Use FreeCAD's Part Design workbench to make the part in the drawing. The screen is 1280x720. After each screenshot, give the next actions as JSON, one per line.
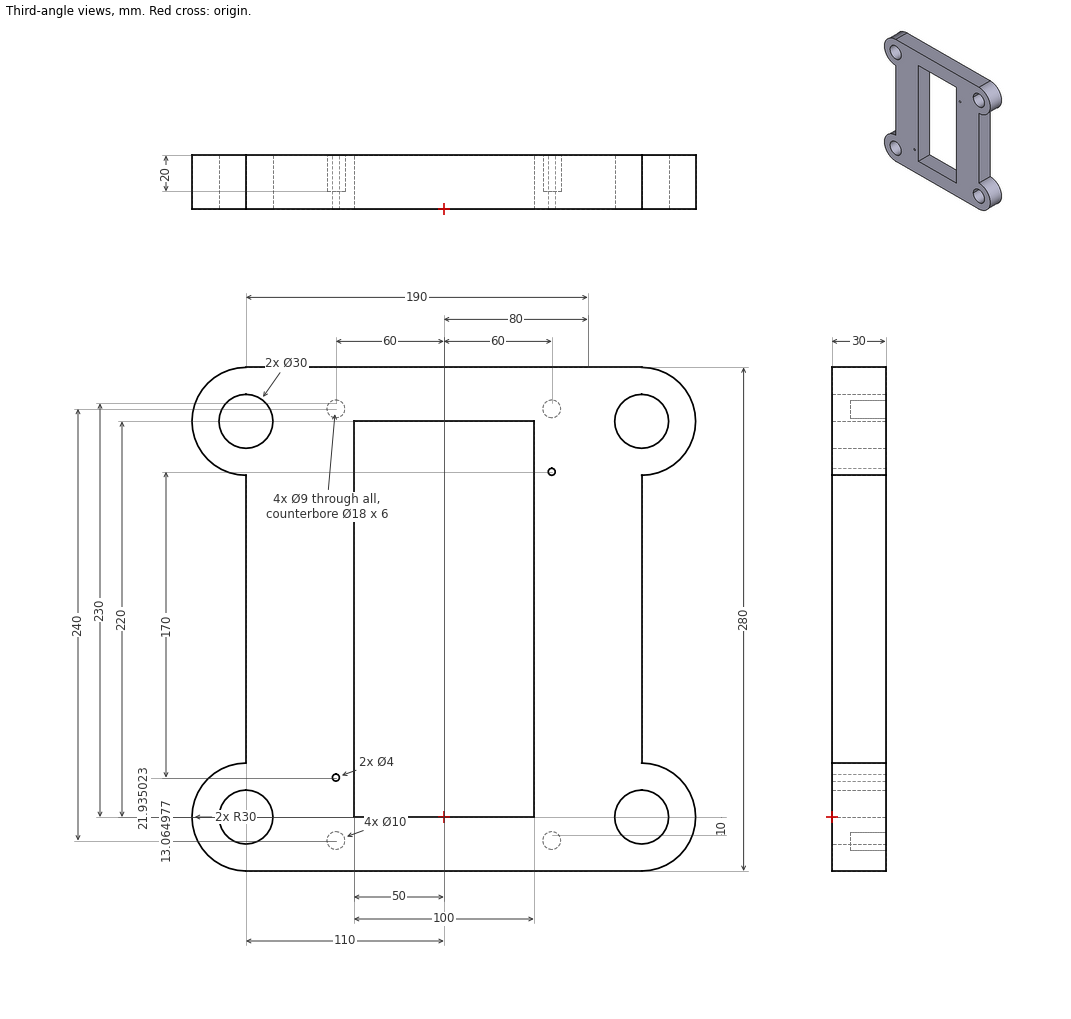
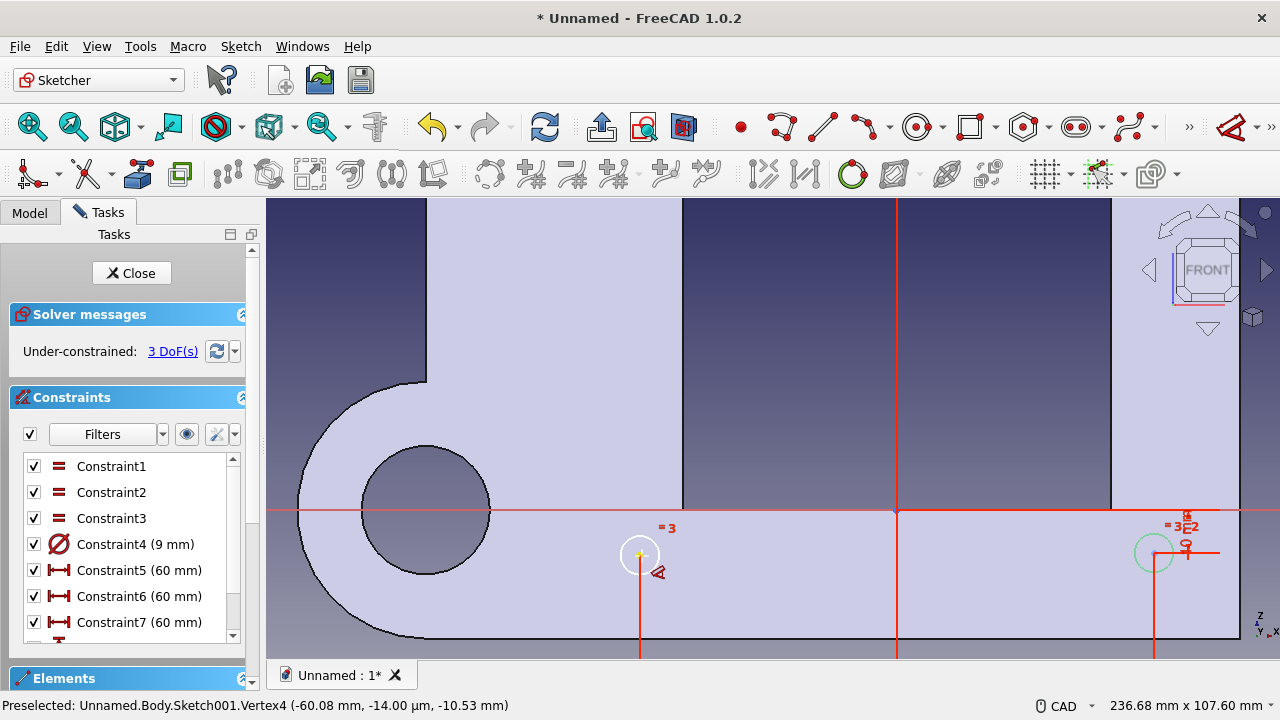
{"action": "left_click", "coordinate": [640, 555]}
{"action": "left_click", "coordinate": [606, 533]}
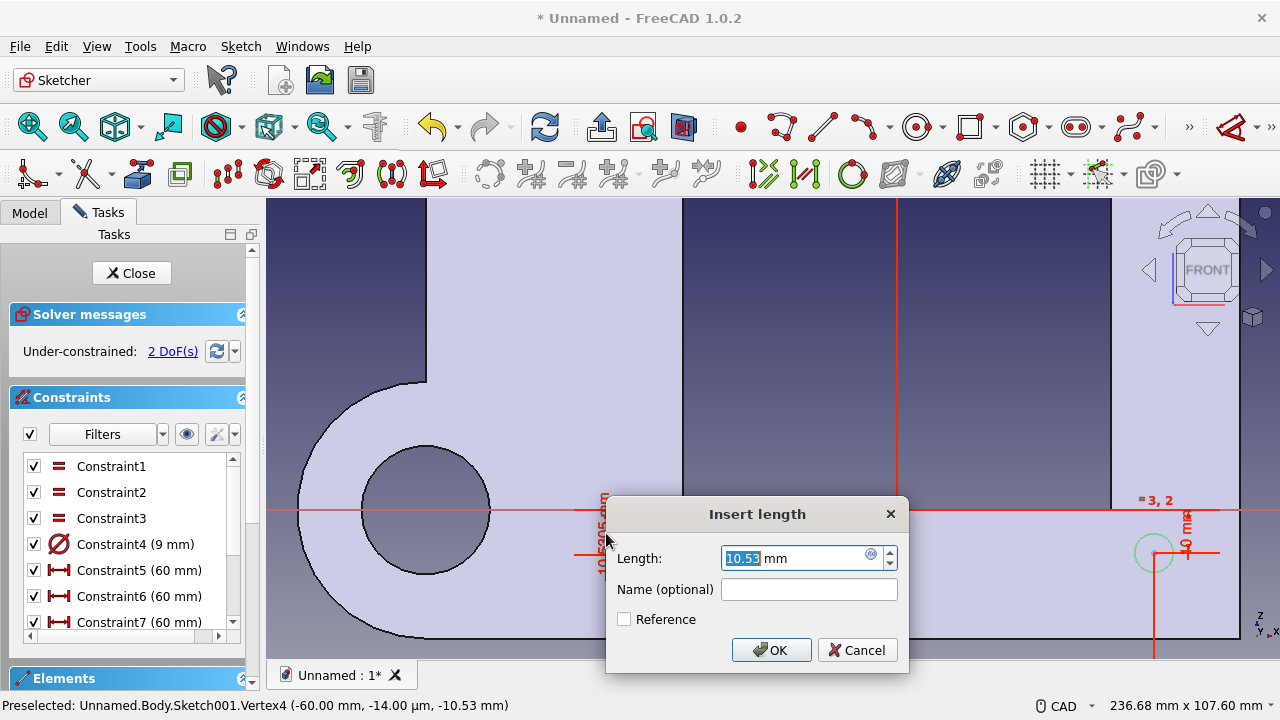
{"action": "type", "text": "10"}
{"action": "key", "text": "Return"}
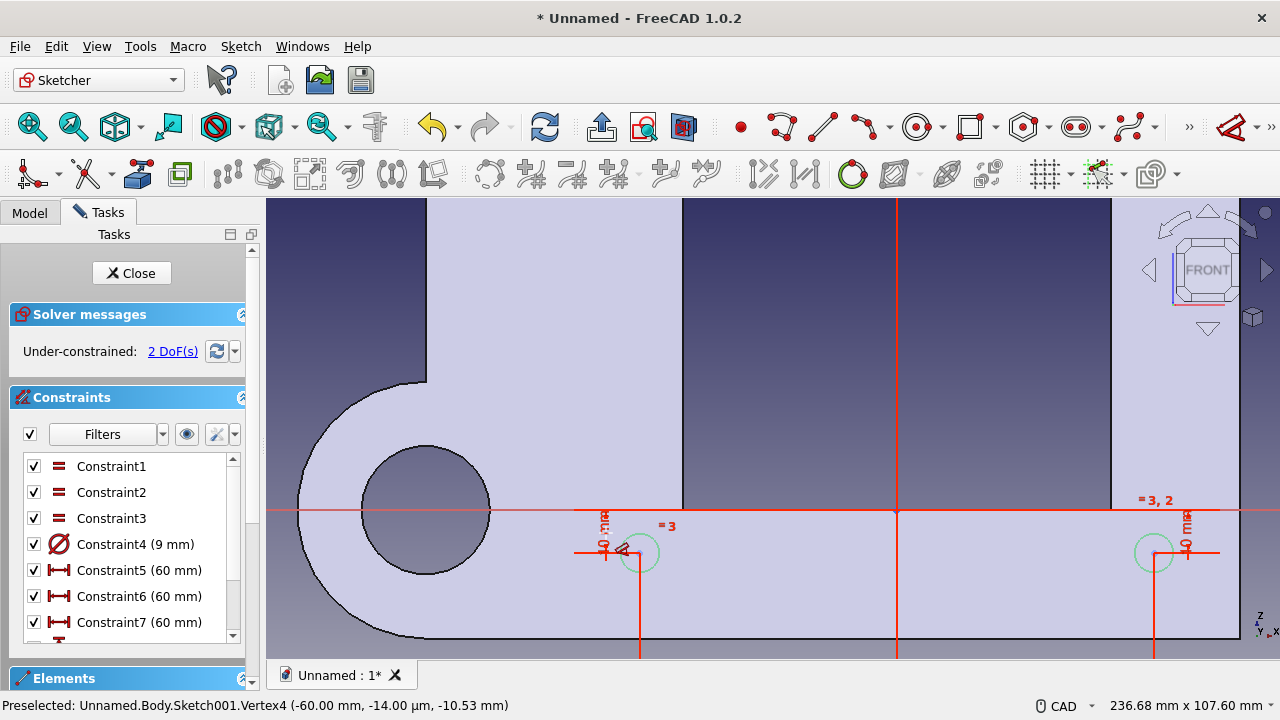
{"action": "scroll", "coordinate": [641, 556], "scroll_direction": "down", "scroll_amount": 7}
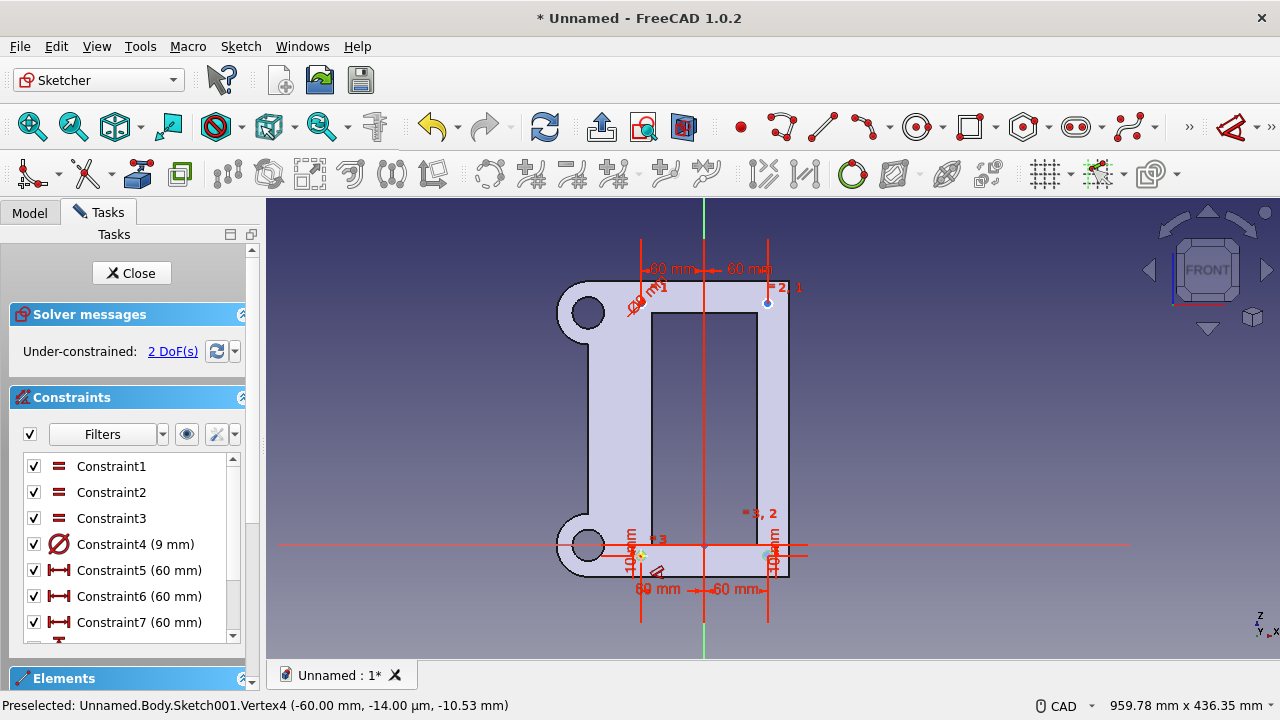
{"action": "left_click", "coordinate": [641, 304]}
{"action": "left_click", "coordinate": [607, 424]}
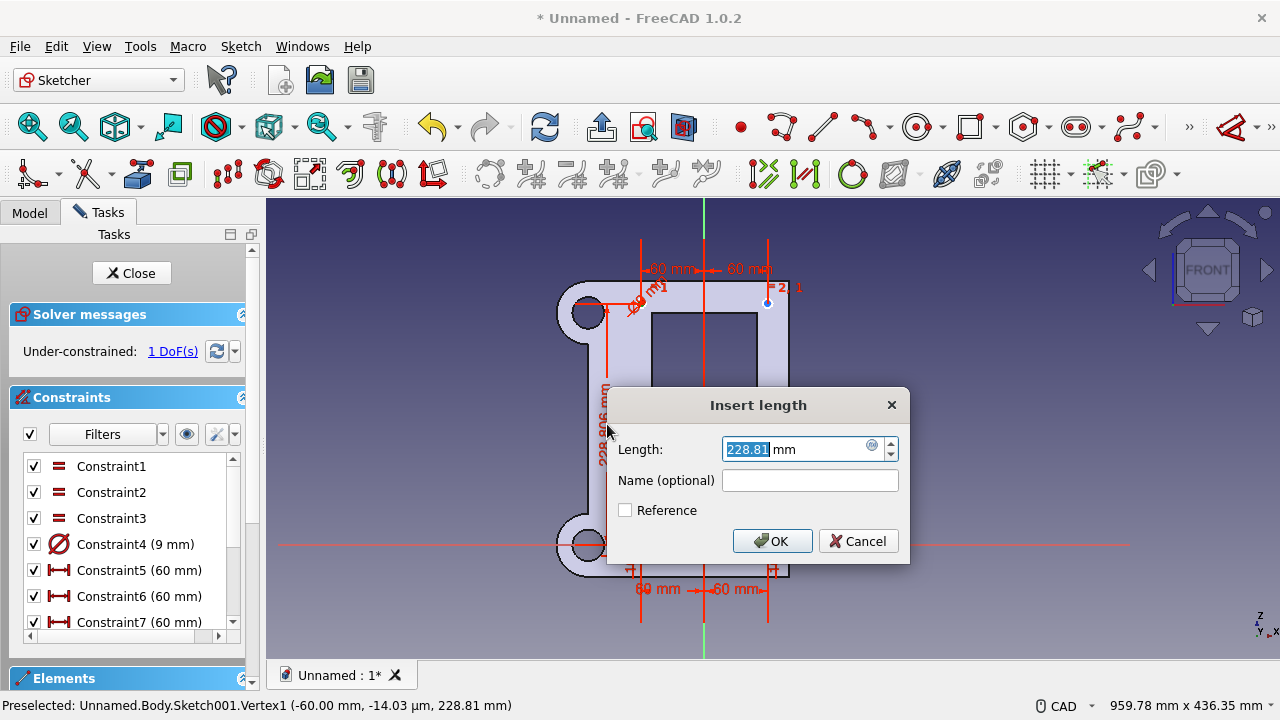
{"action": "type", "text": "230"}
{"action": "key", "text": "Return"}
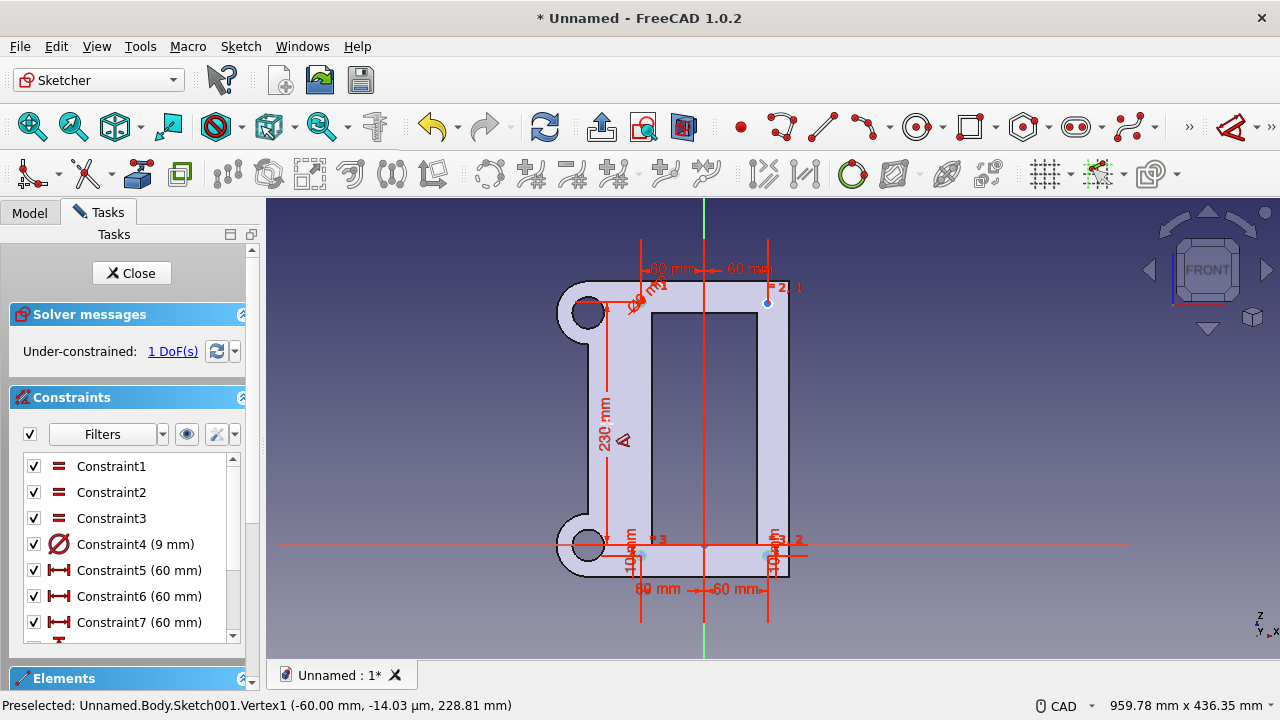
{"action": "left_click", "coordinate": [768, 304]}
{"action": "left_click", "coordinate": [802, 424]}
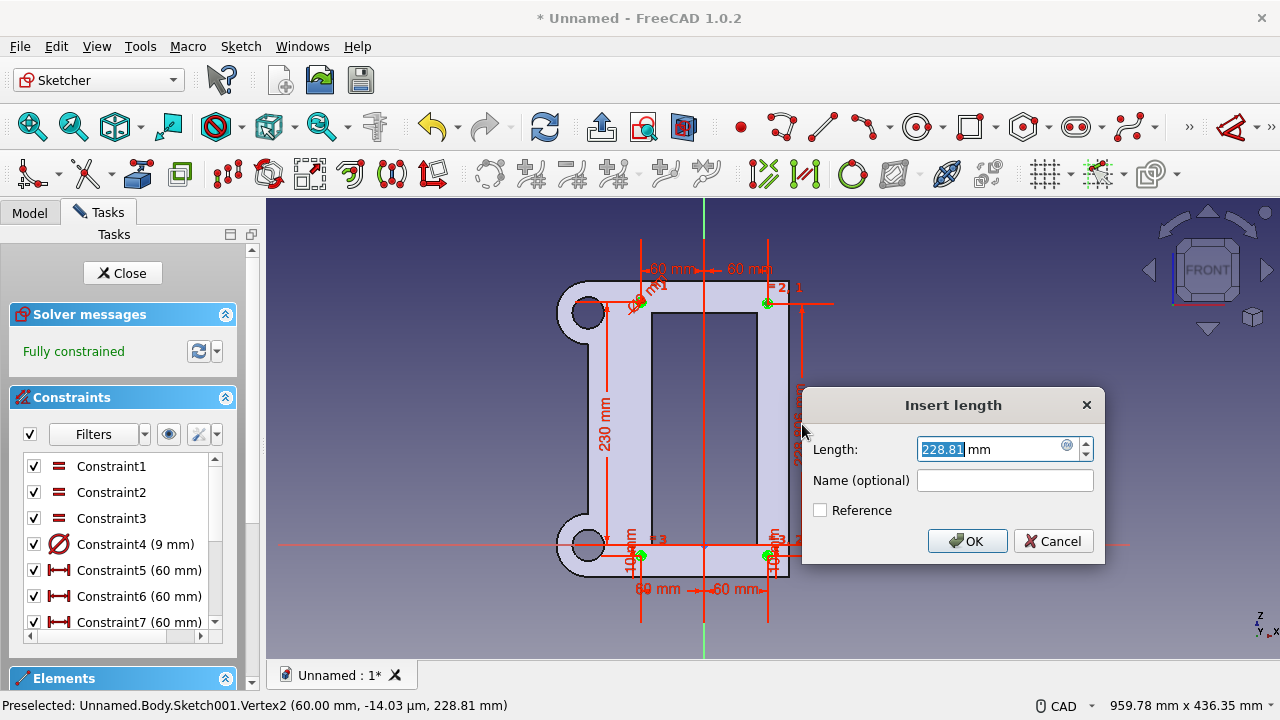
{"action": "type", "text": "230"}
{"action": "key", "text": "Return"}
{"action": "key", "text": "Escape"}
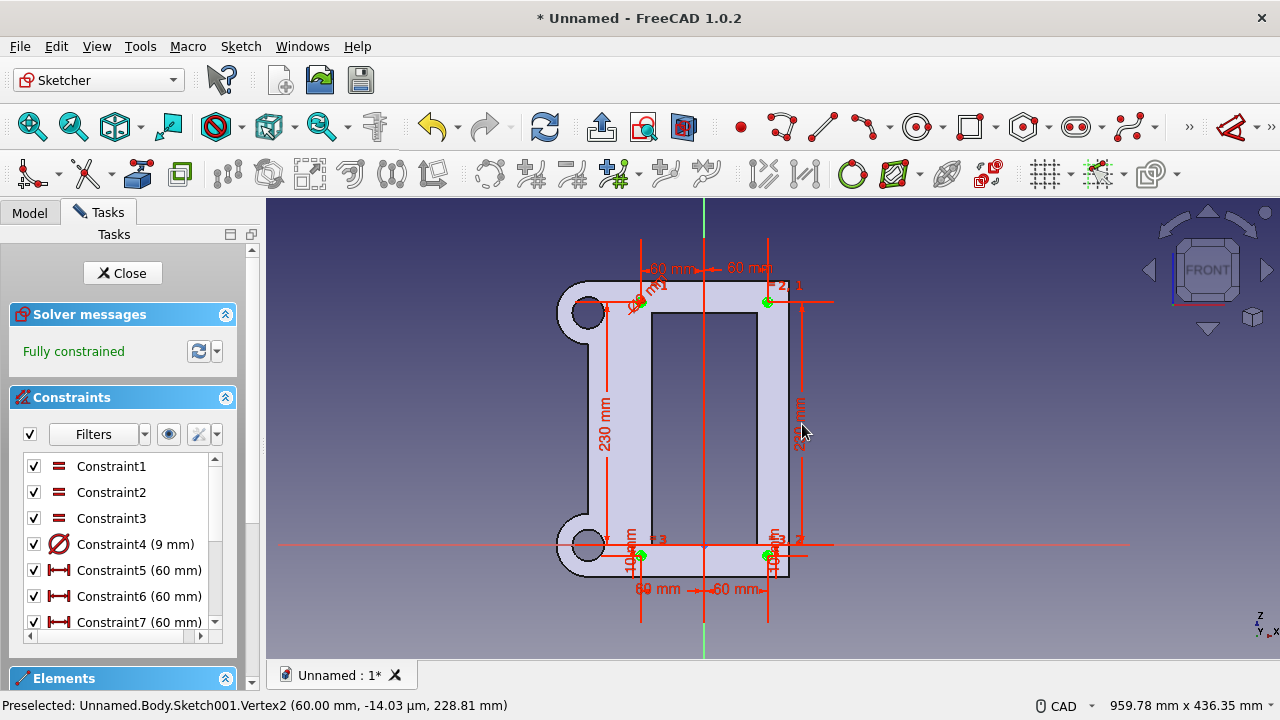
{"action": "left_click", "coordinate": [123, 273]}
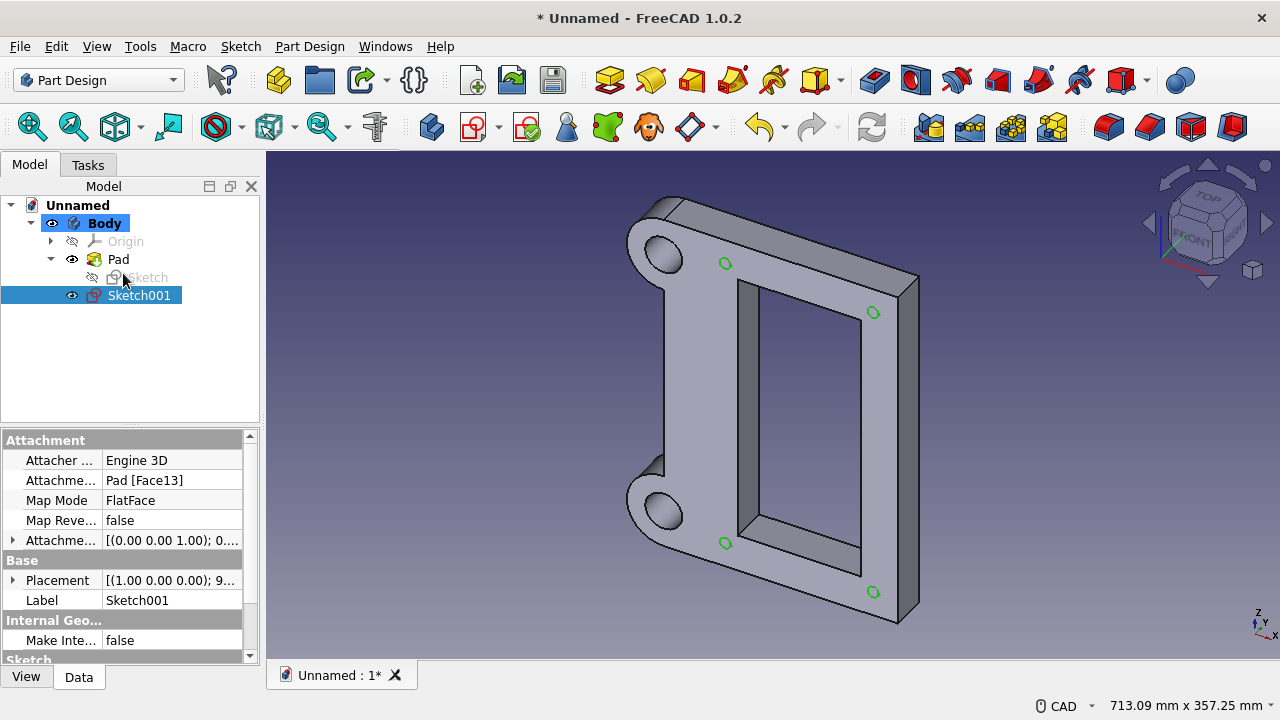
{"action": "left_click", "coordinate": [916, 80]}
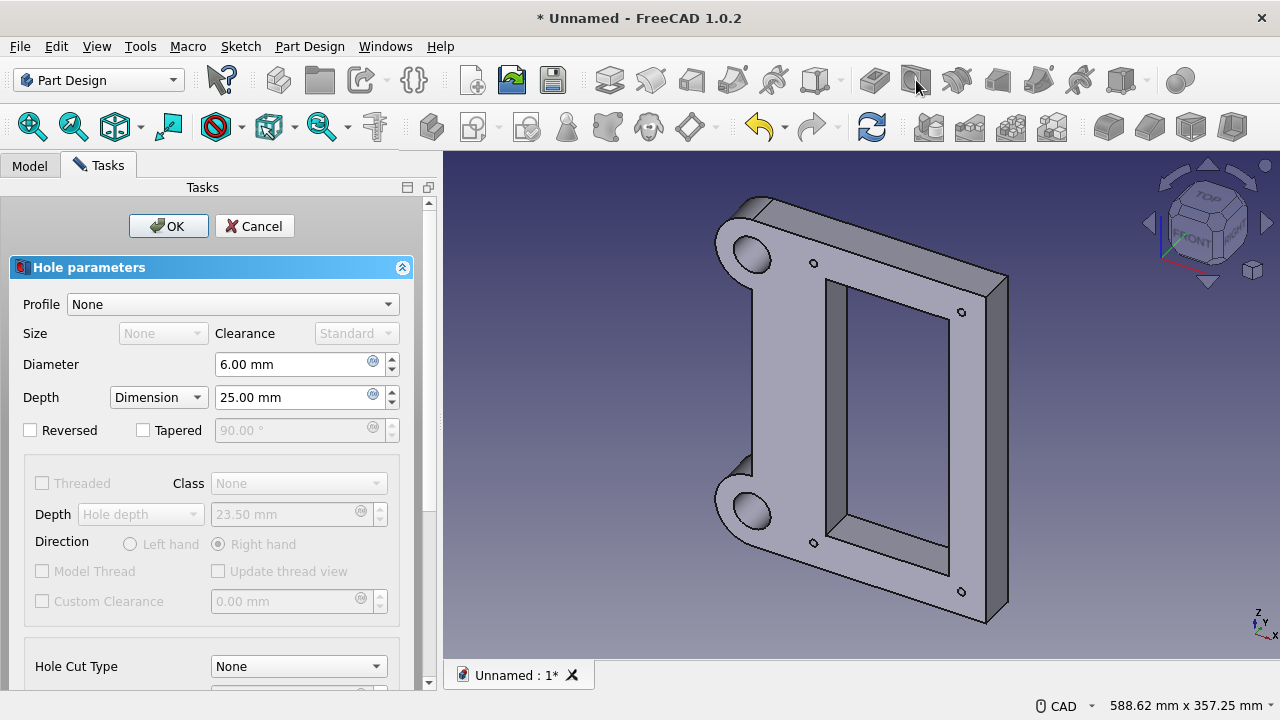
{"action": "triple_click", "coordinate": [300, 364]}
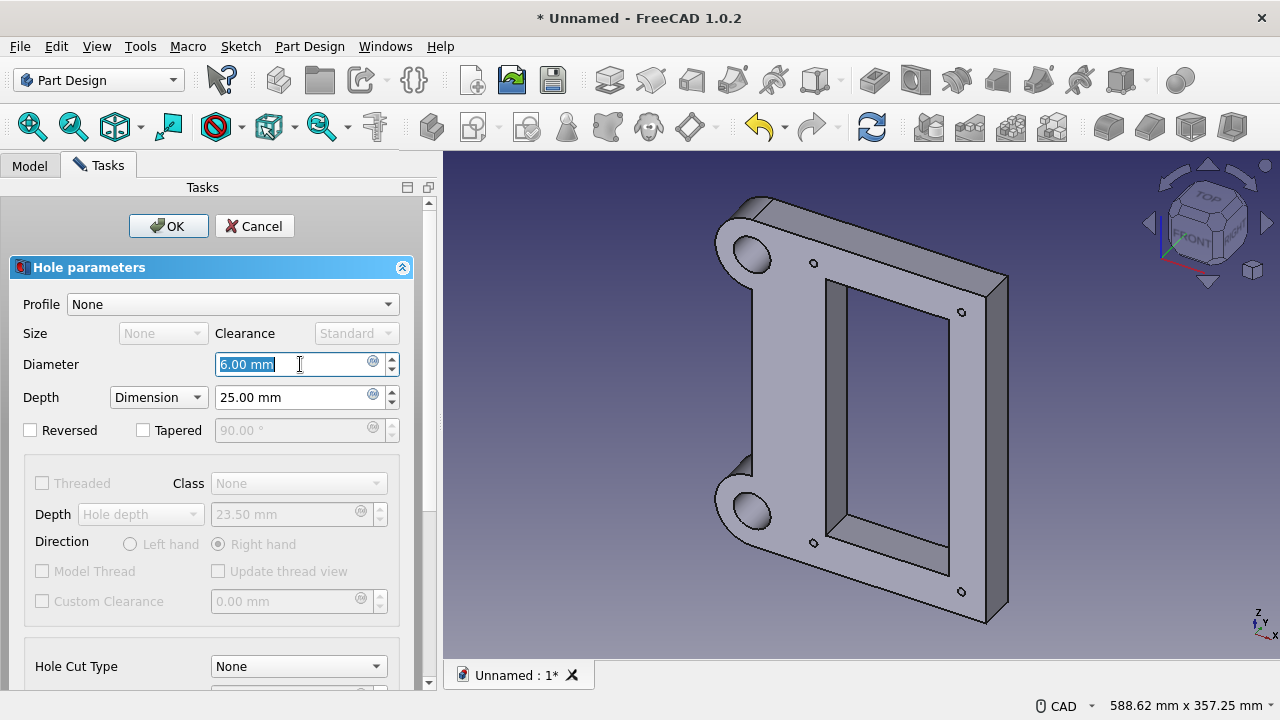
{"action": "type", "text": "9"}
{"action": "key", "text": "Tab"}